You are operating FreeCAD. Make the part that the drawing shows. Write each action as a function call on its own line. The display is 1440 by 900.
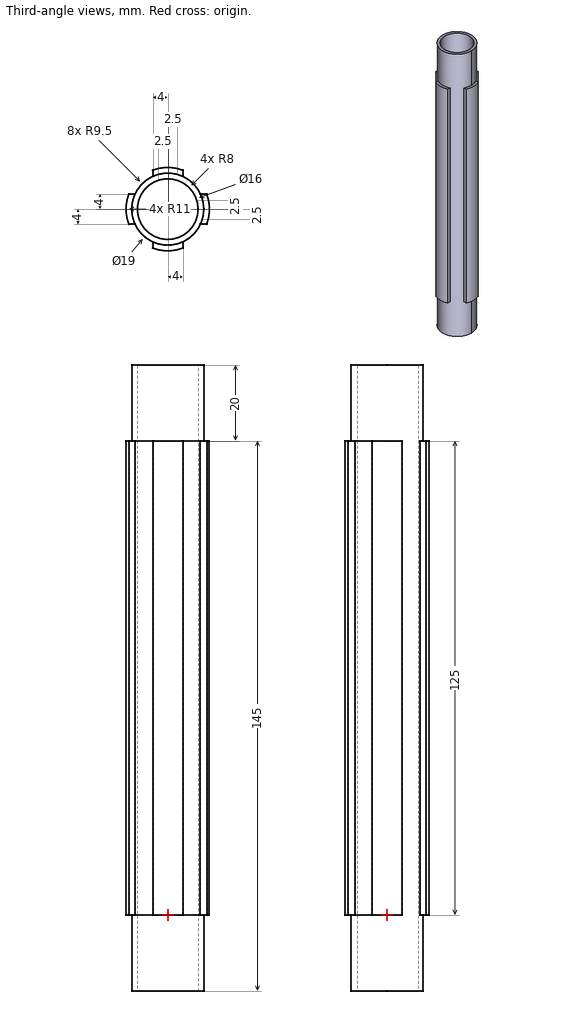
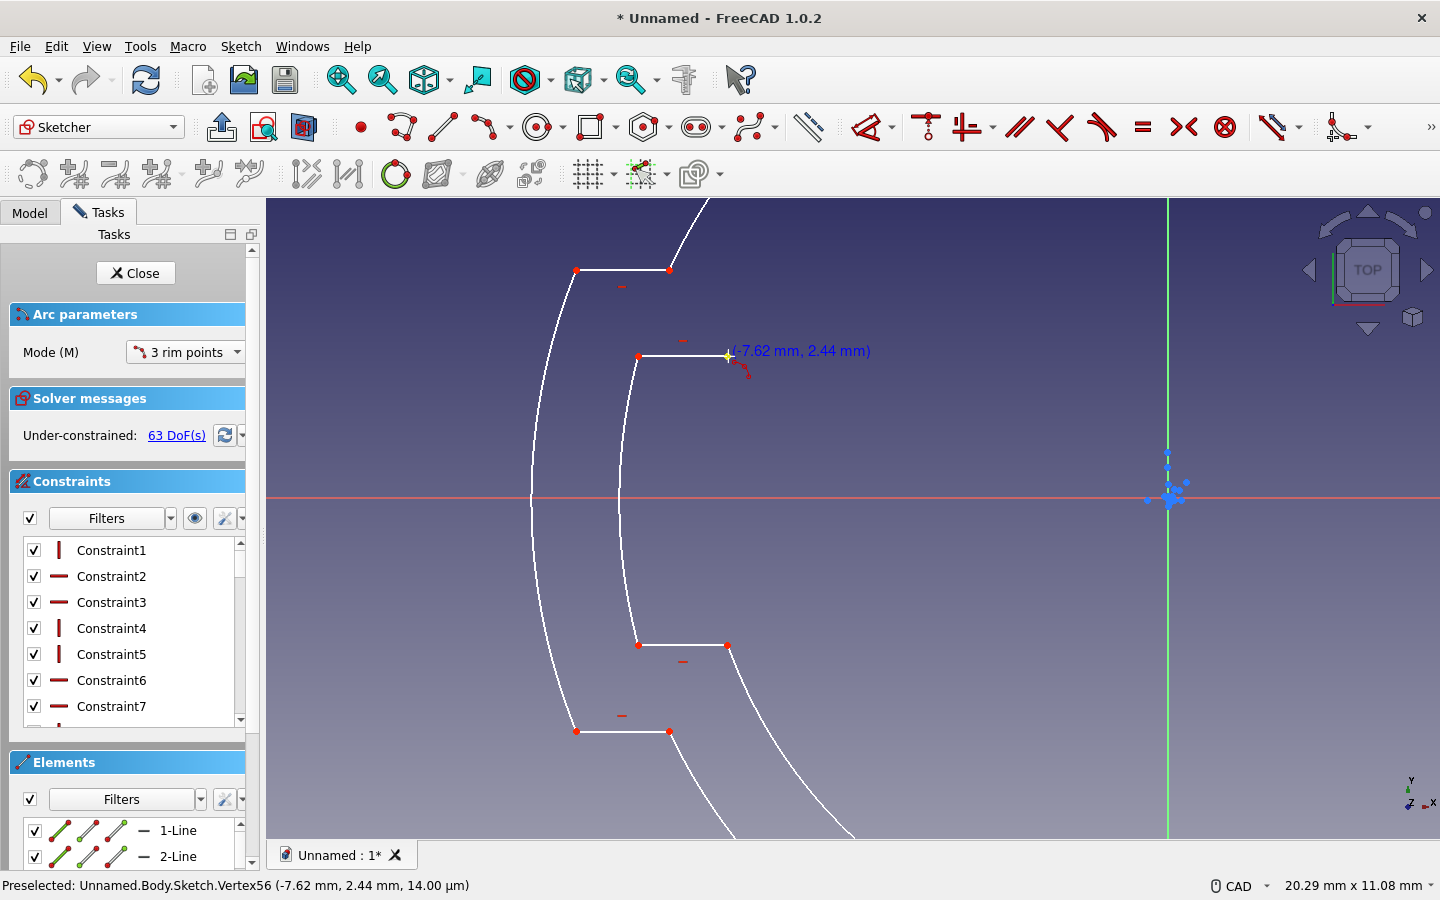
scroll(619, 528, down, 6)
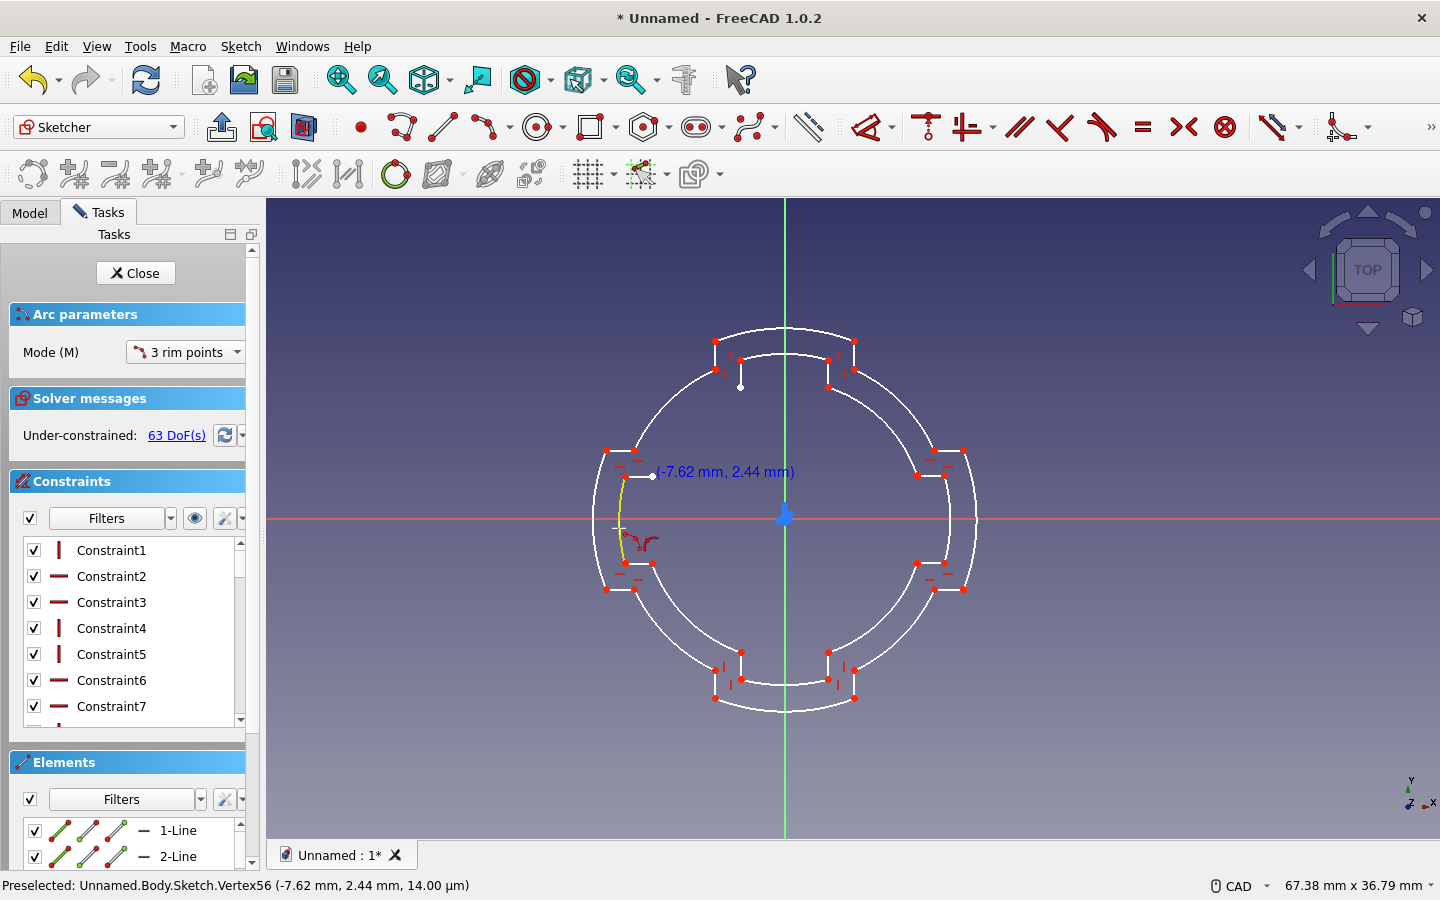
click(741, 388)
click(686, 421)
key(Escape)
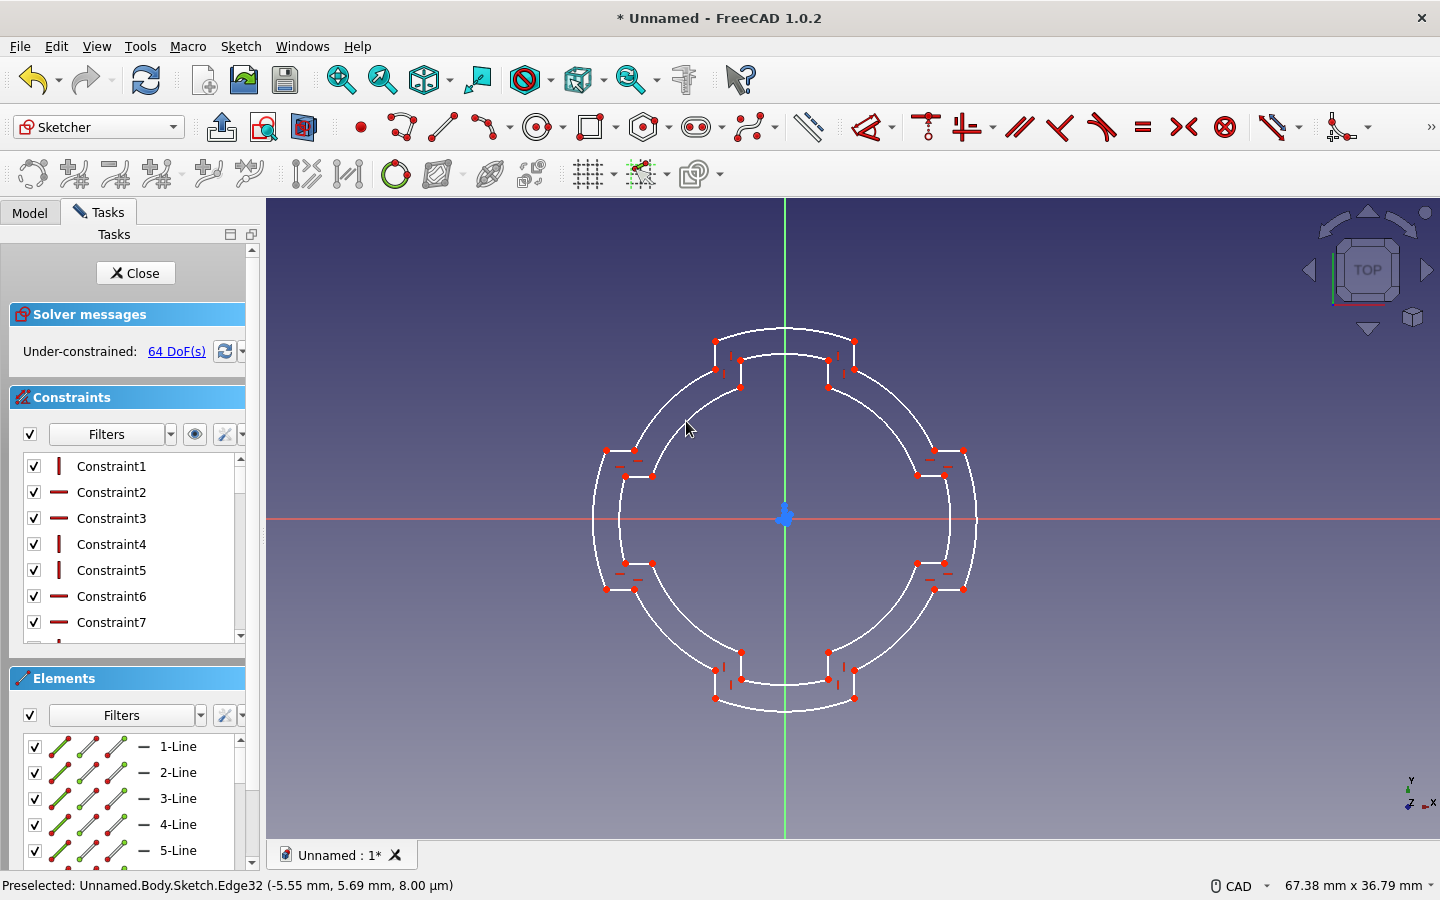
click(685, 388)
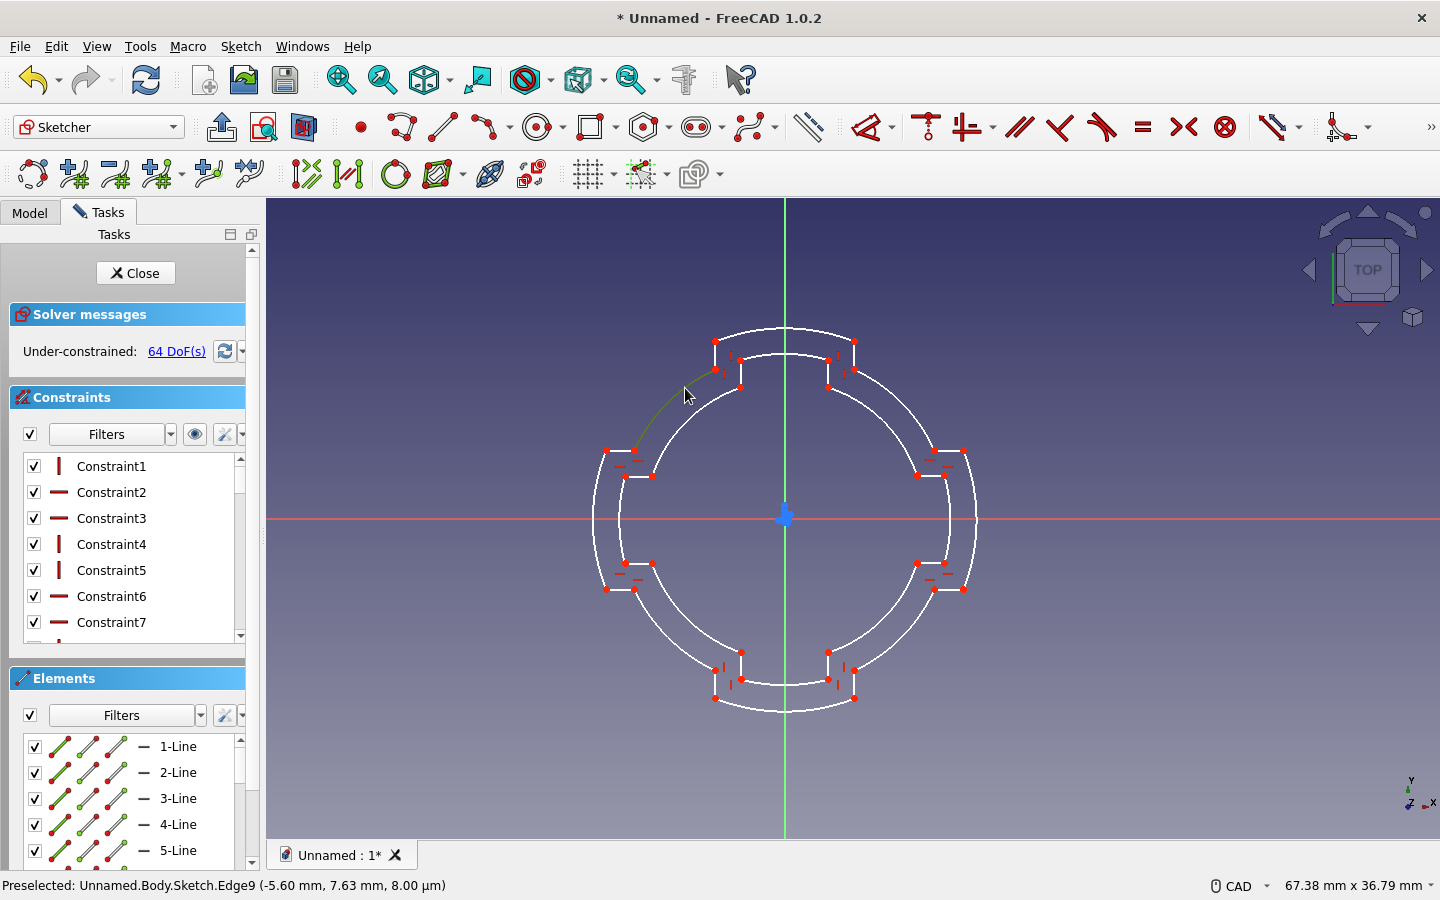
click(595, 492)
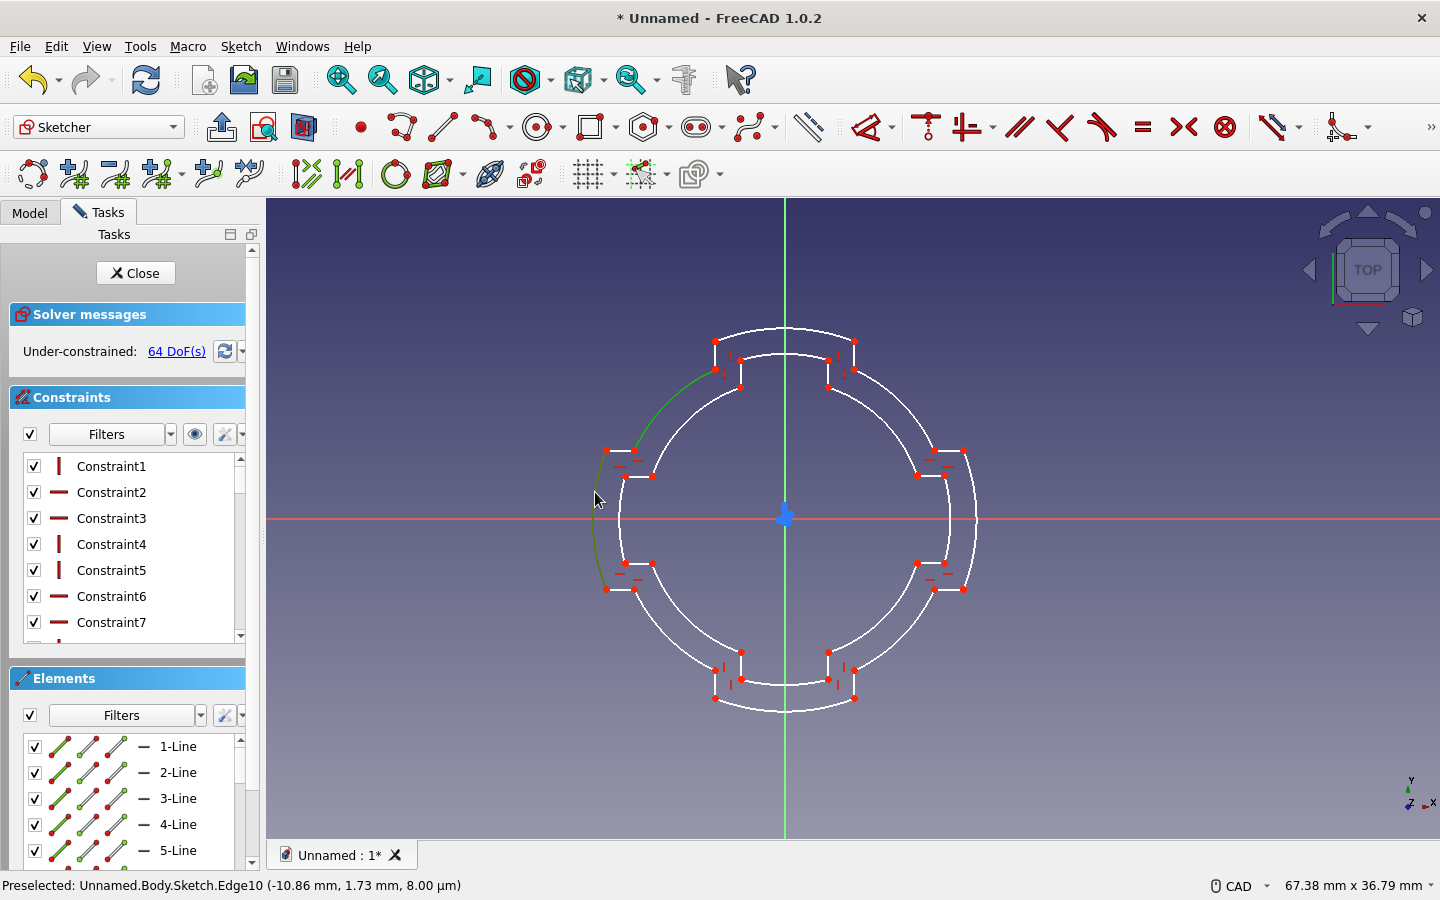
click(926, 128)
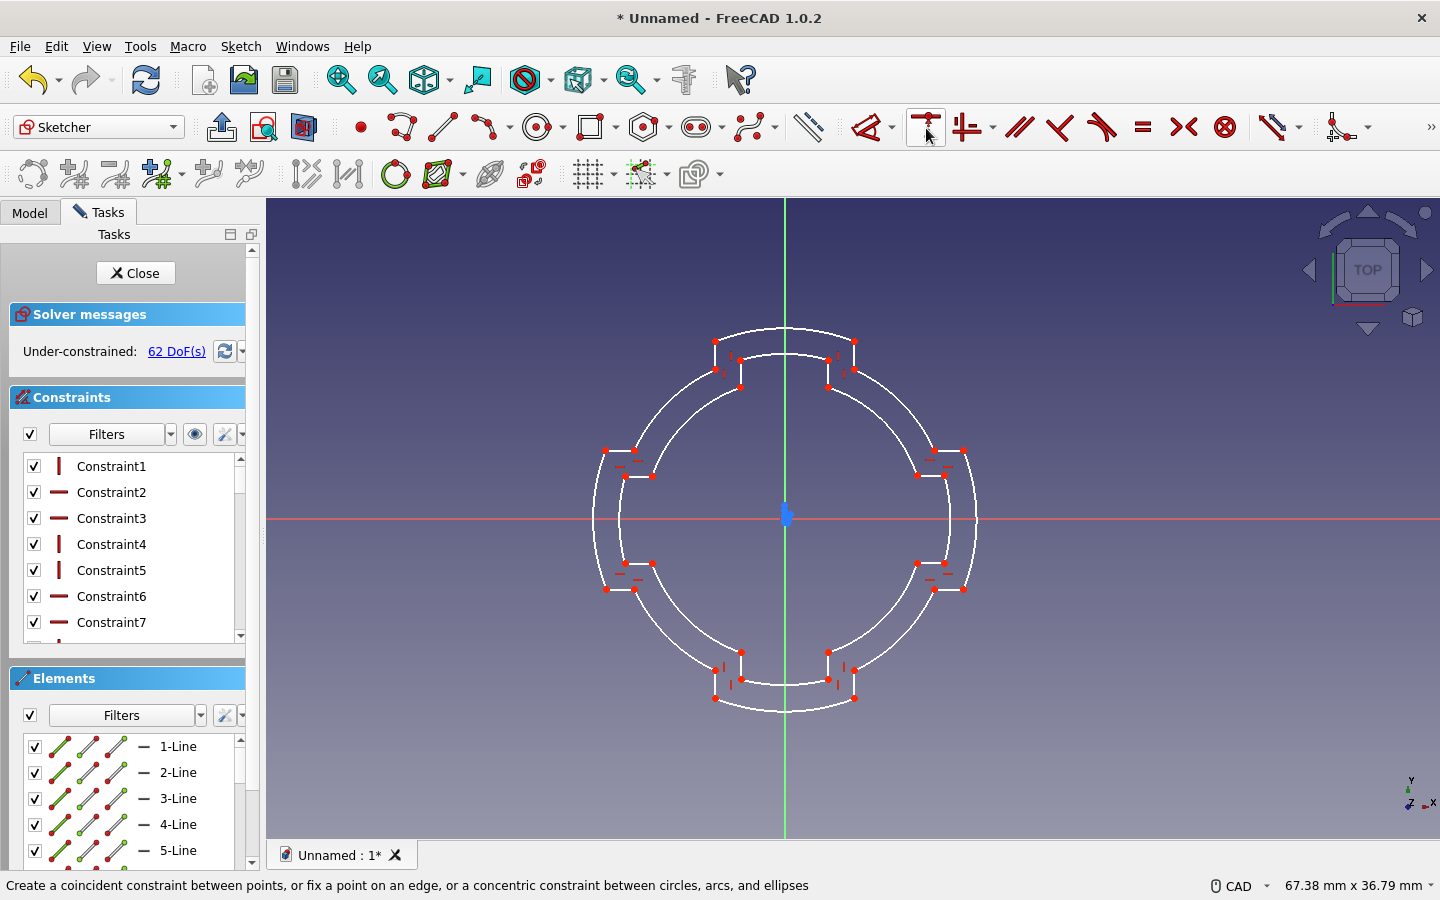
click(685, 388)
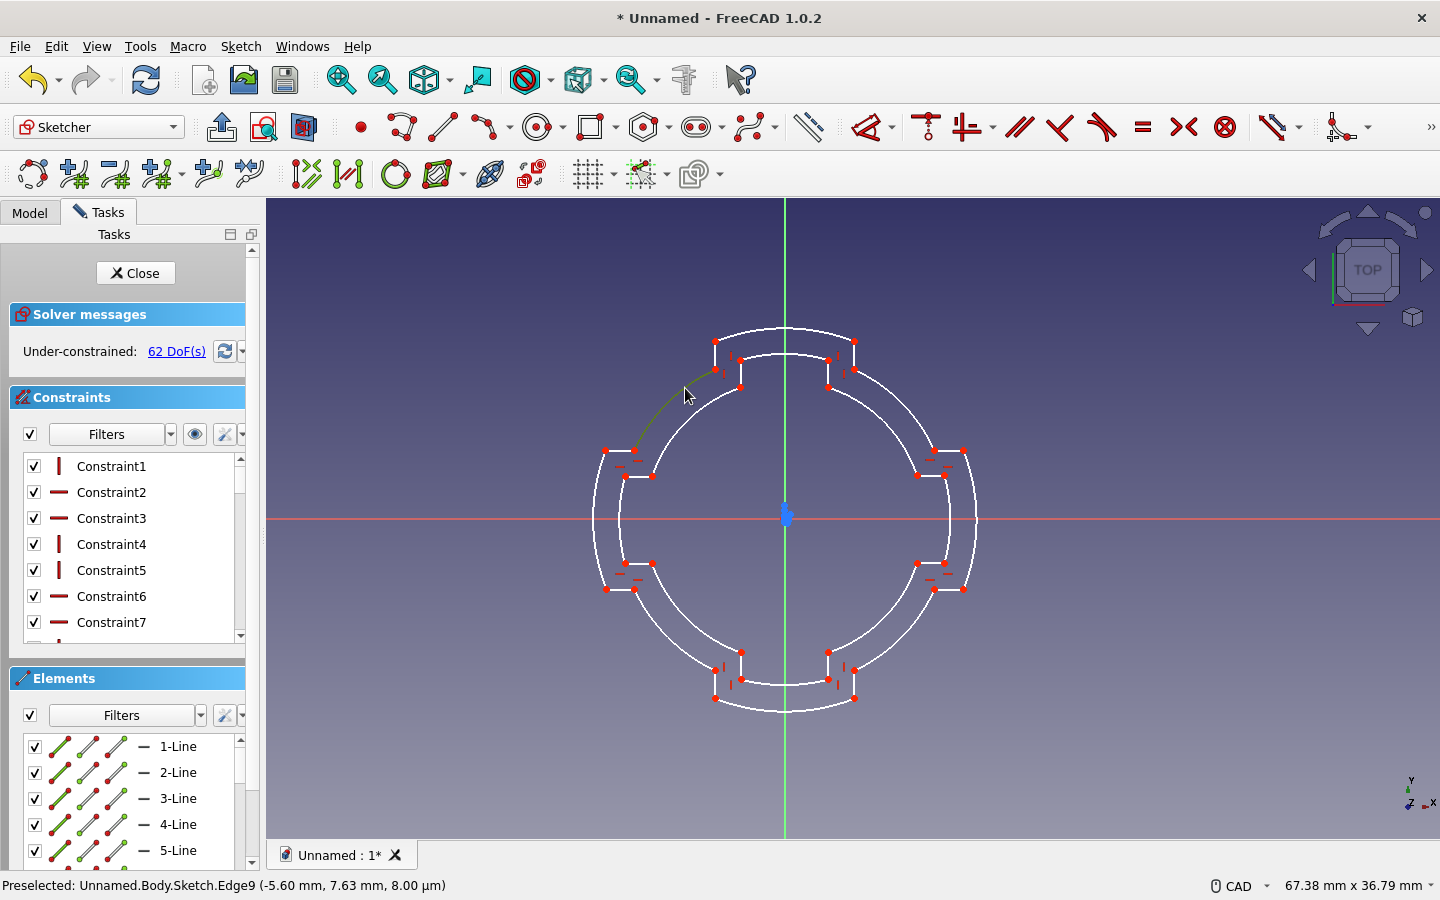
click(652, 620)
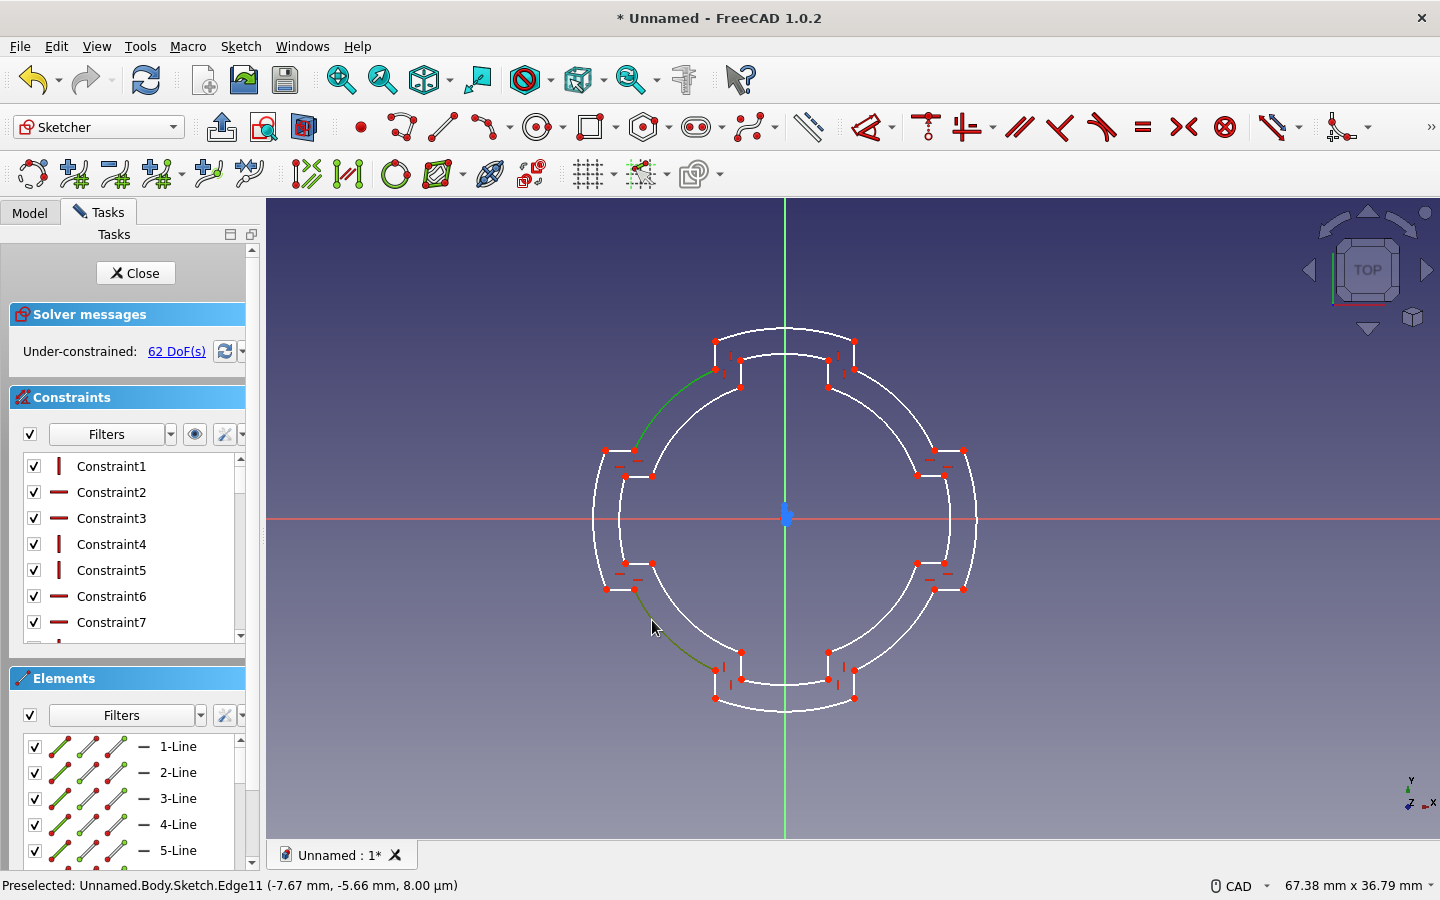
click(926, 128)